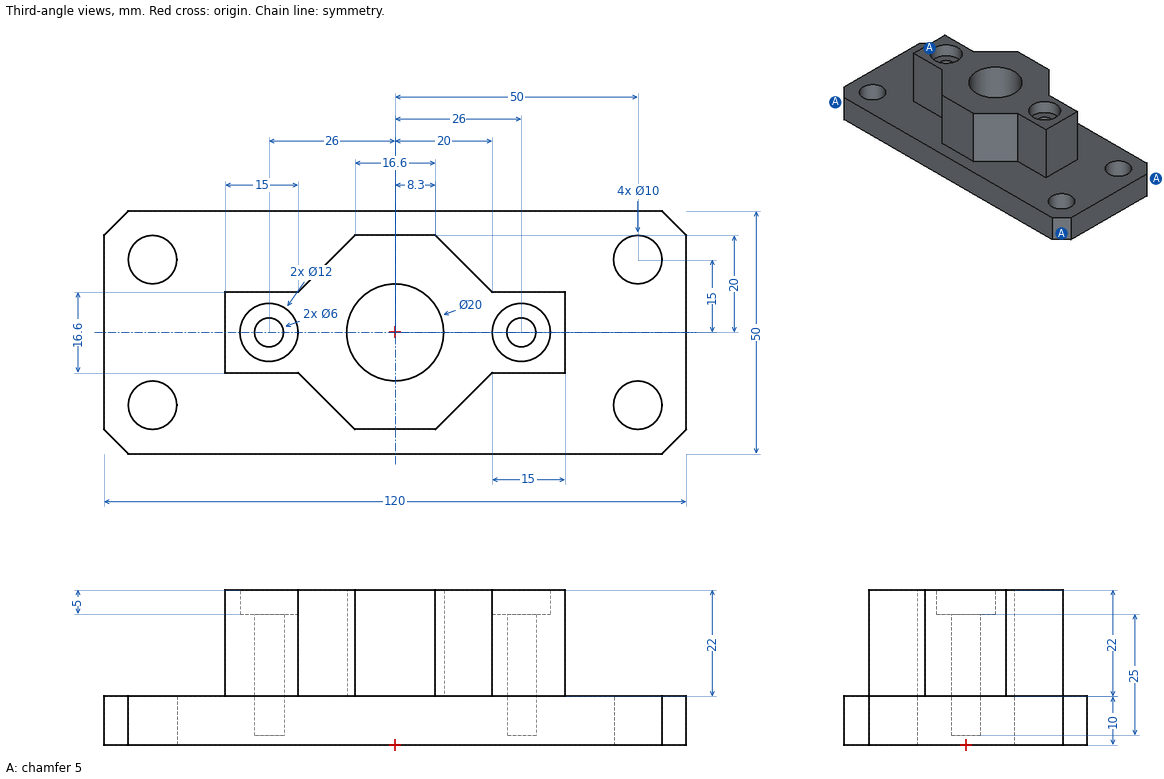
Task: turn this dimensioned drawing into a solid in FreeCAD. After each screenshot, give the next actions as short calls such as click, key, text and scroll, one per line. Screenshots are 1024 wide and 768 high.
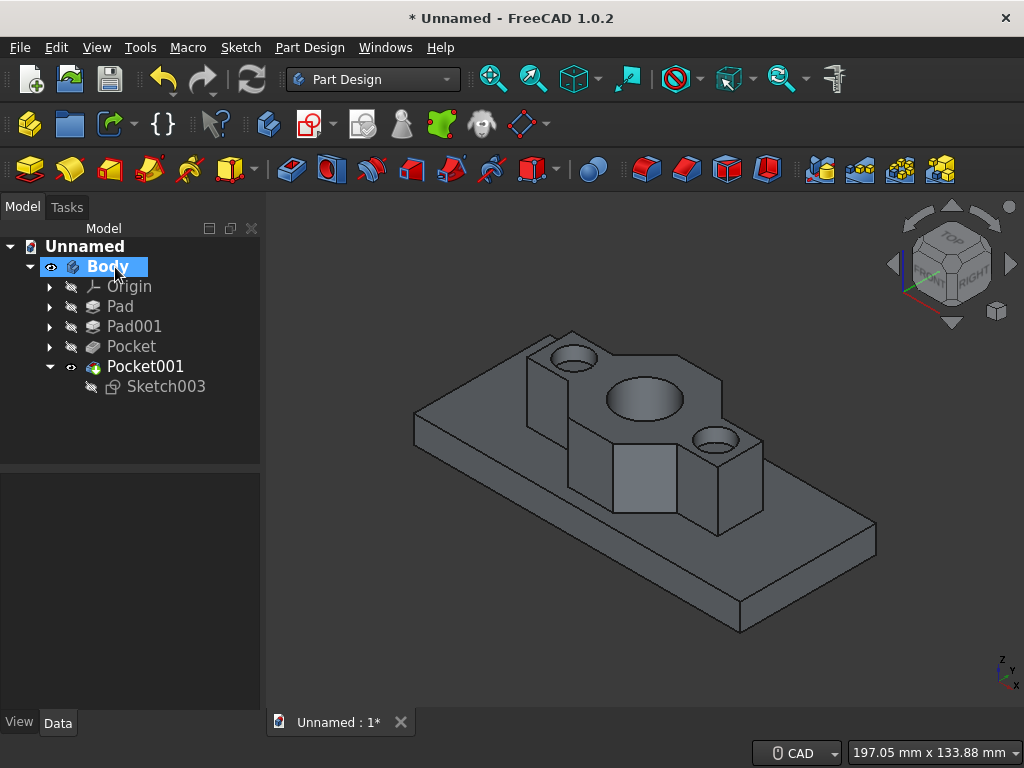
key(2)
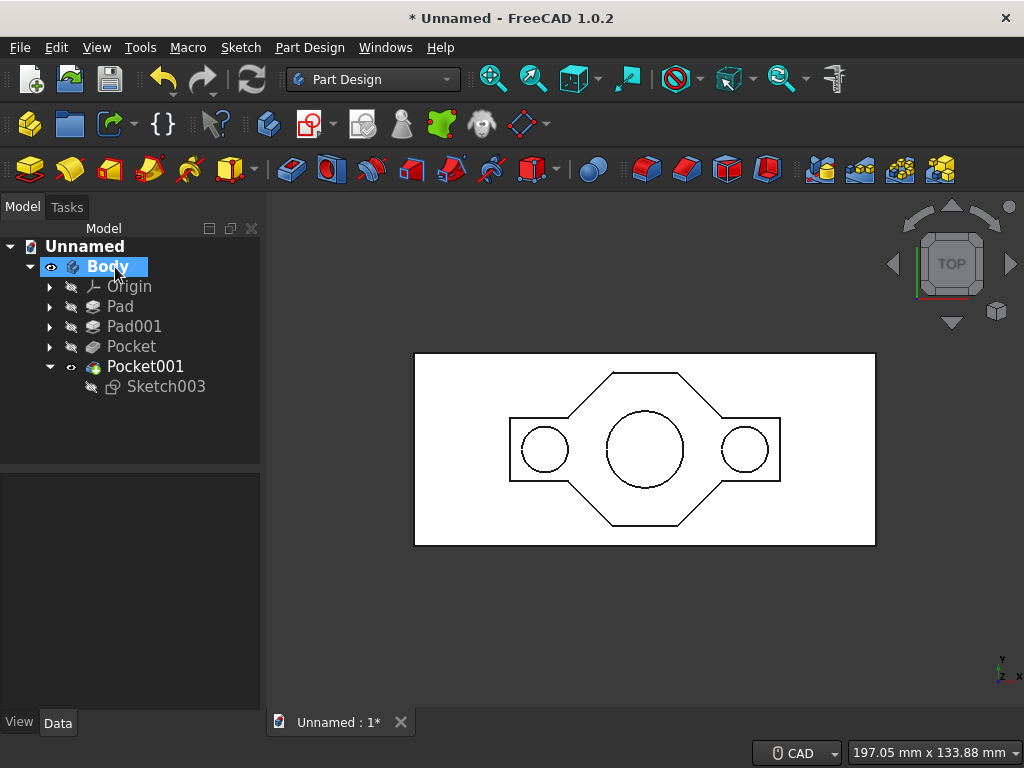
click(745, 449)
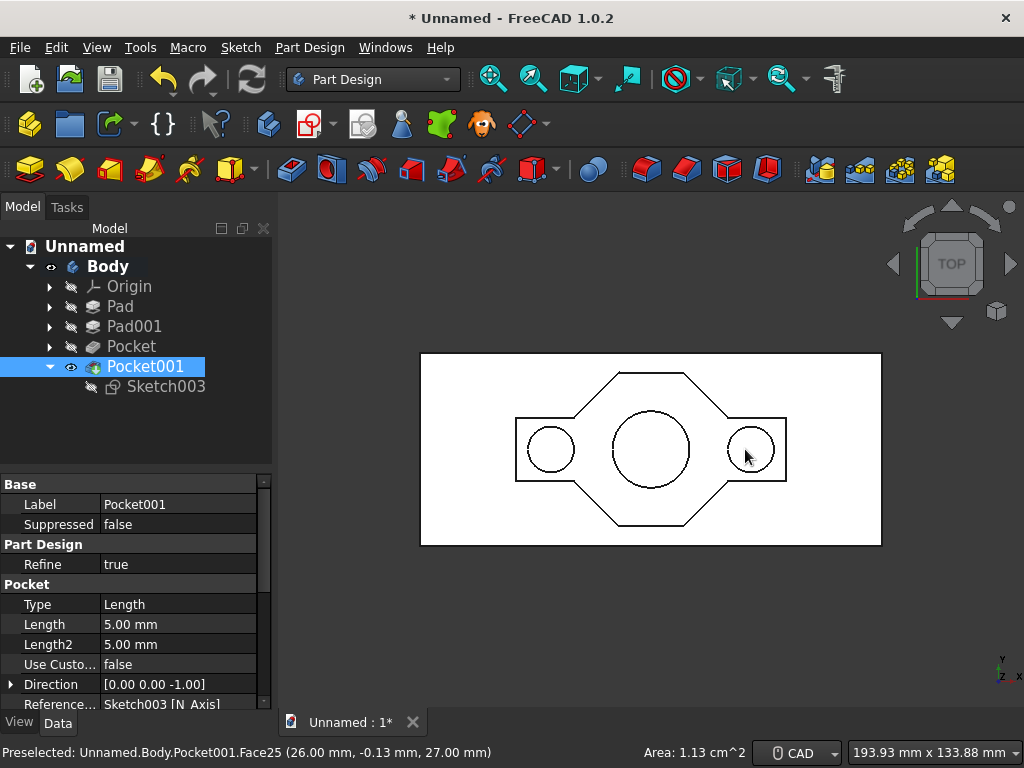
click(310, 124)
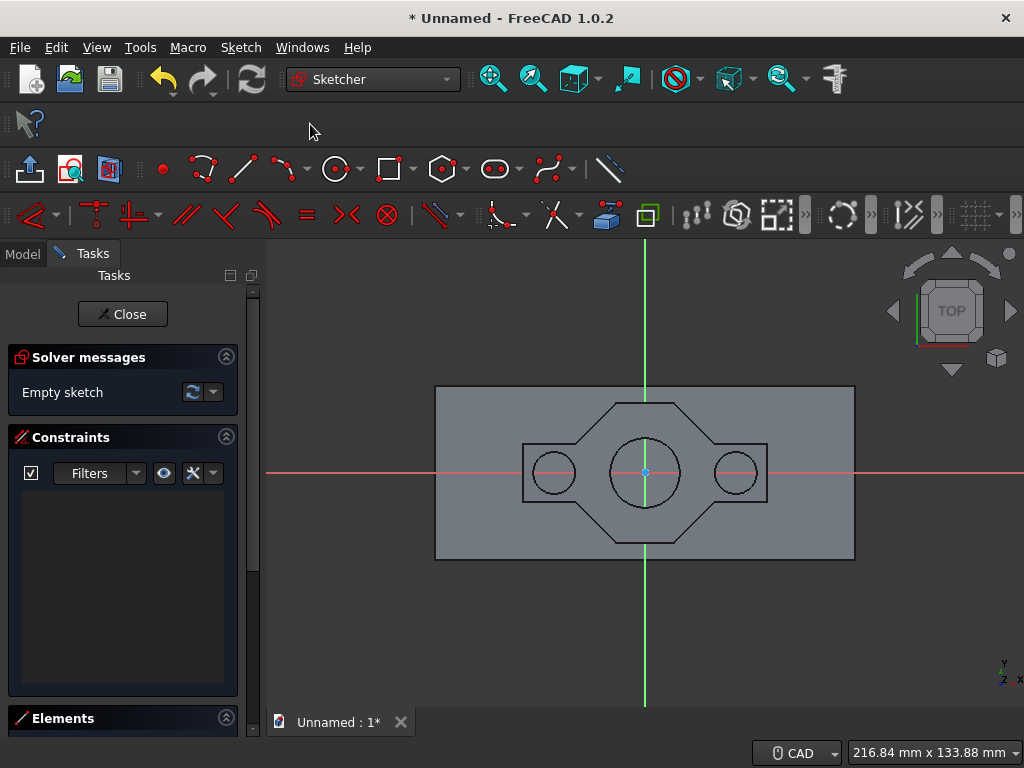
click(110, 170)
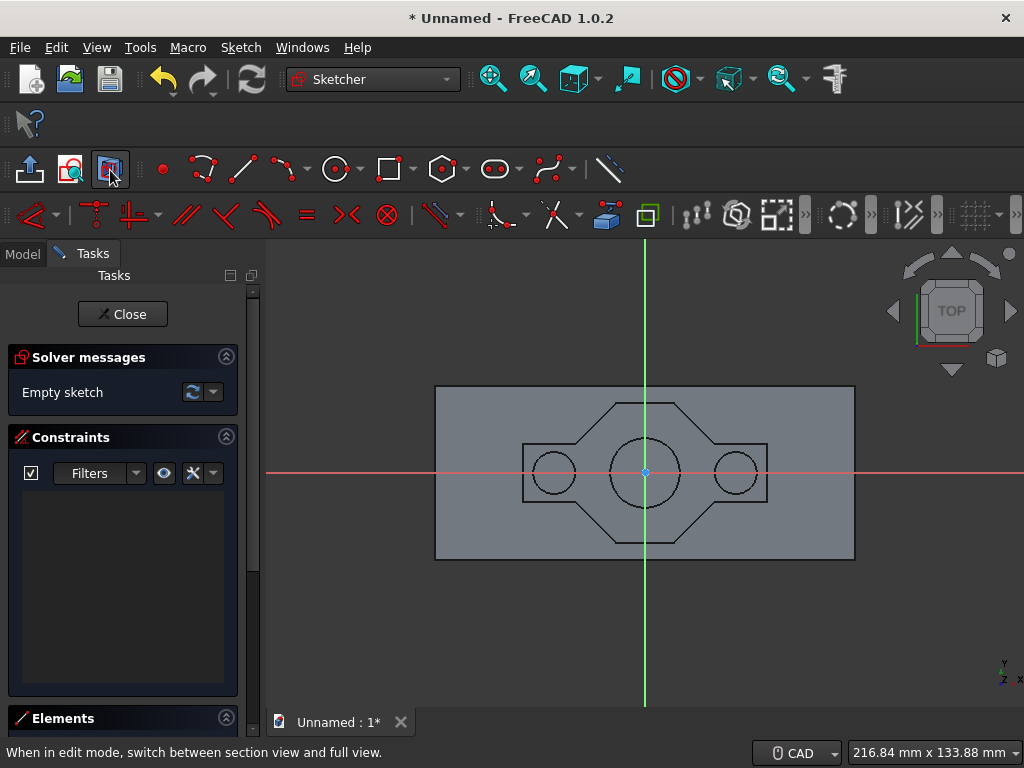
scroll(728, 473, up, 3)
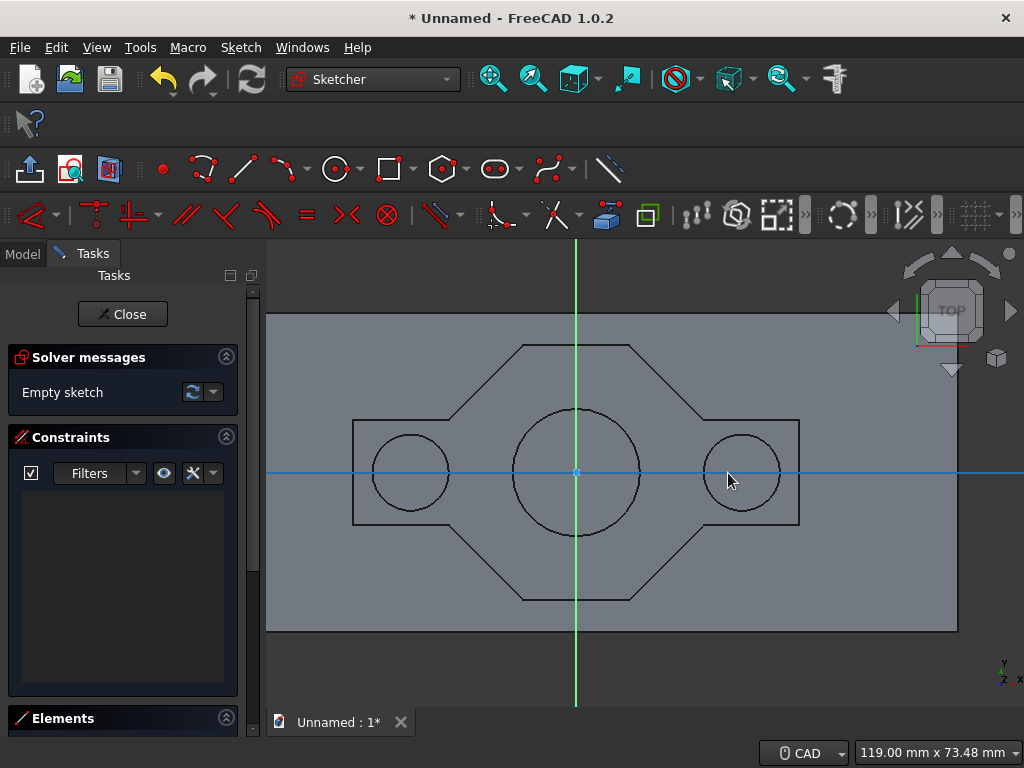
click(336, 170)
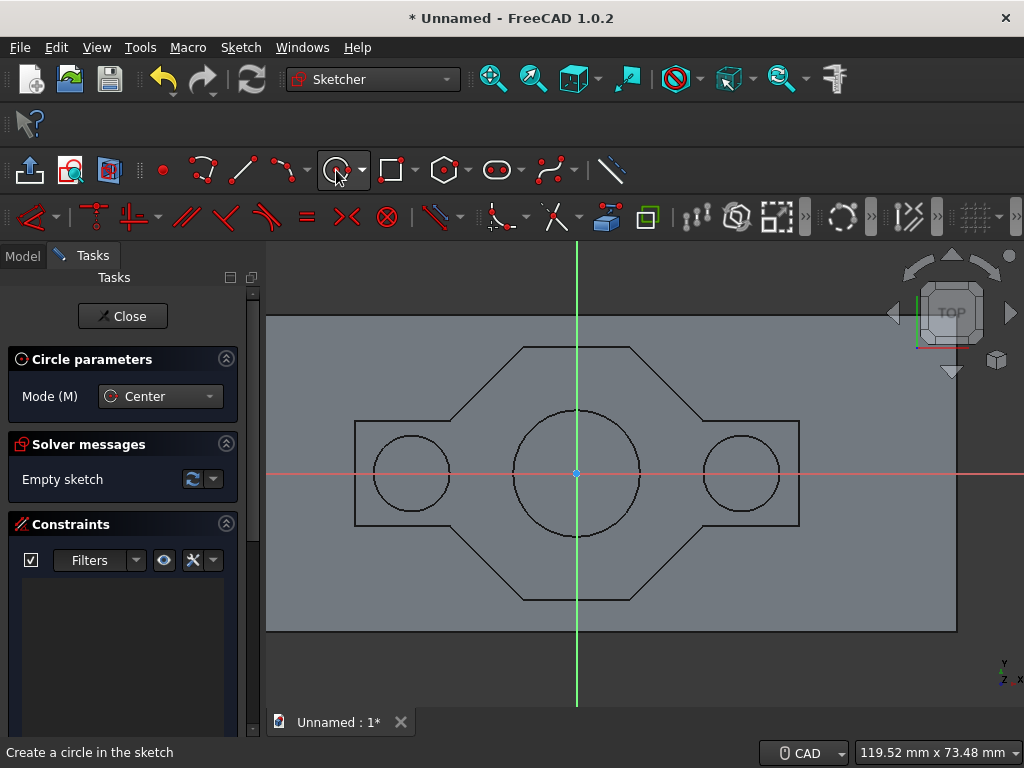
click(412, 474)
click(418, 456)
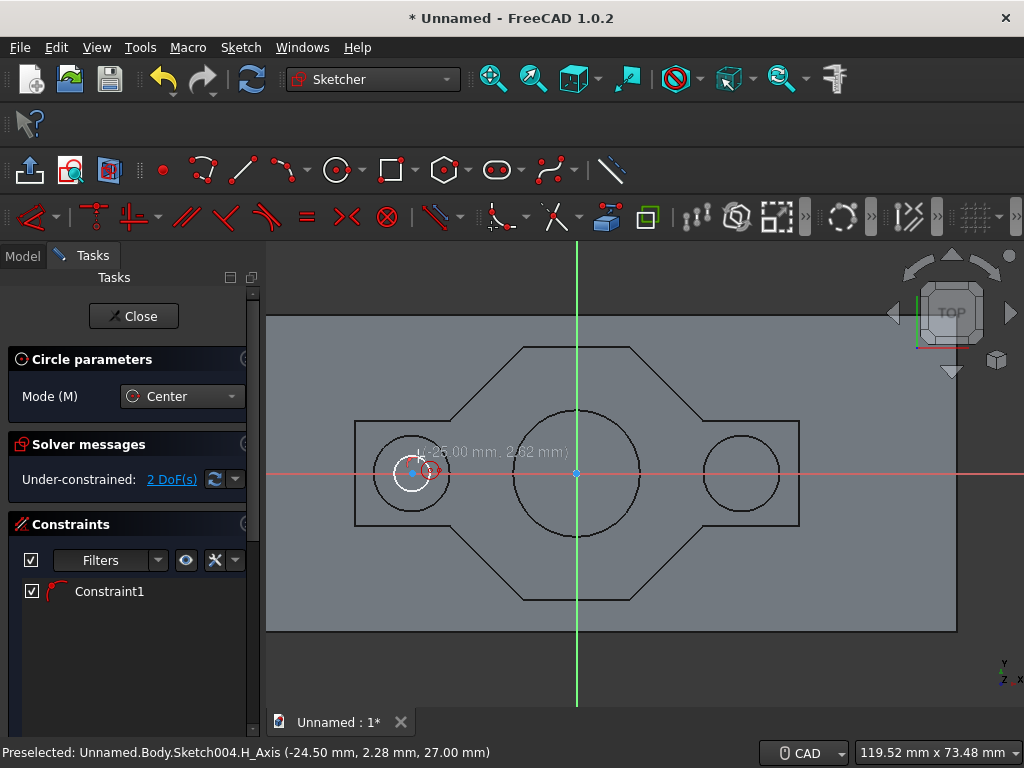
click(741, 474)
click(748, 456)
key(Escape)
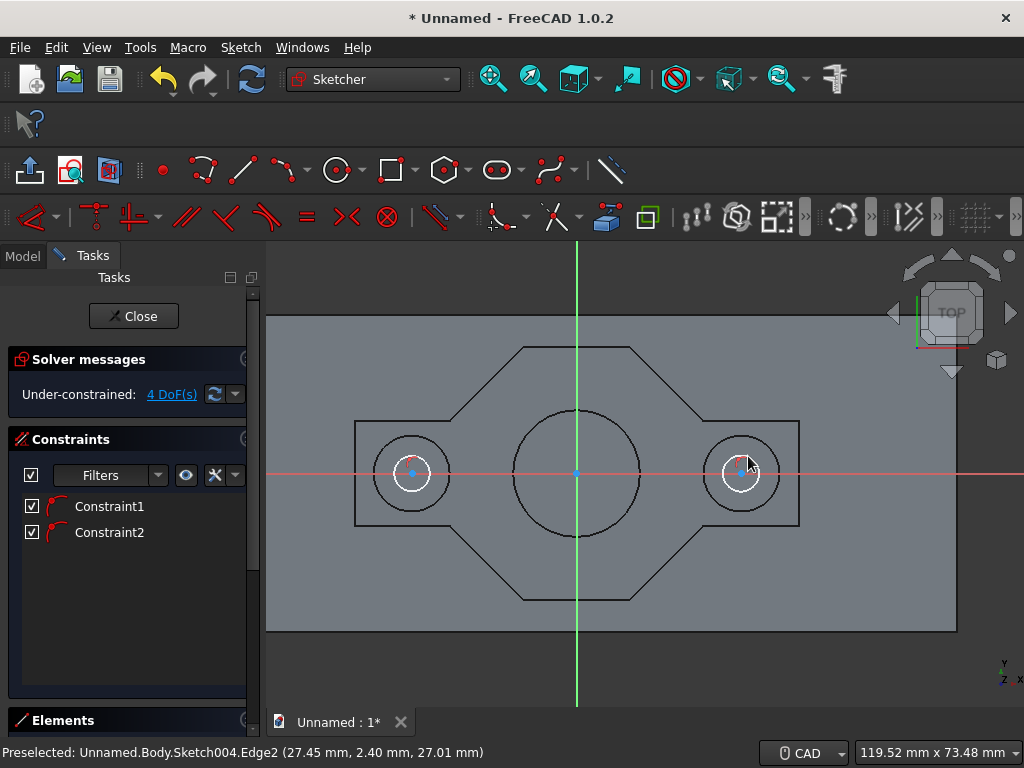
click(424, 461)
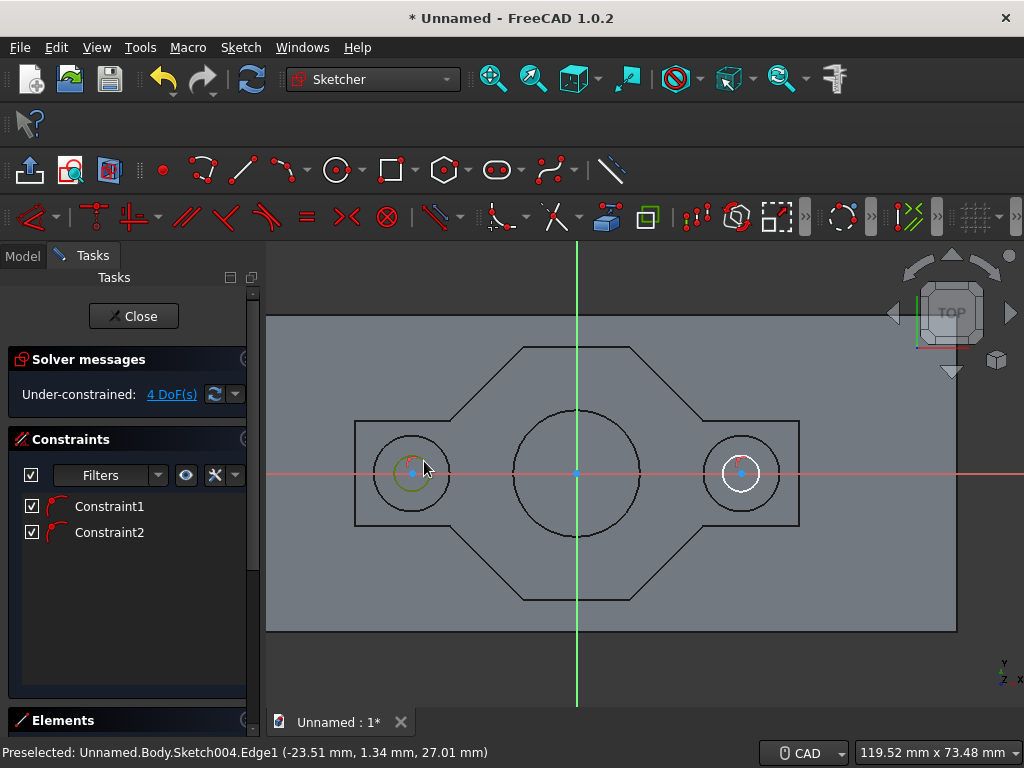
click(754, 461)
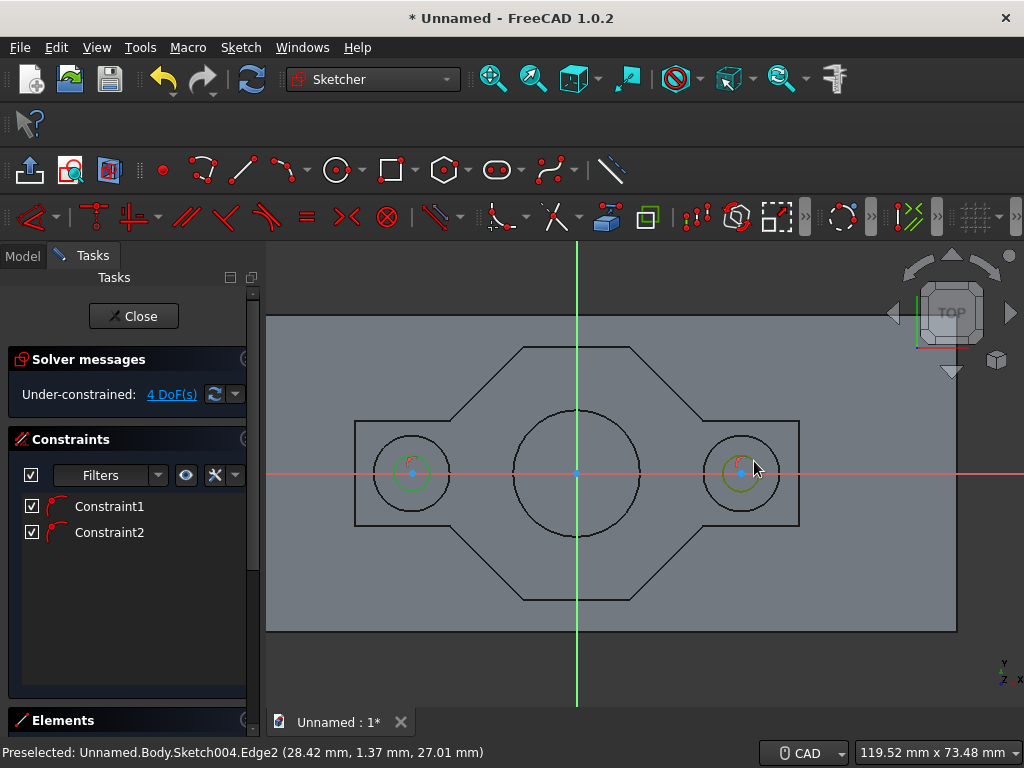
click(308, 218)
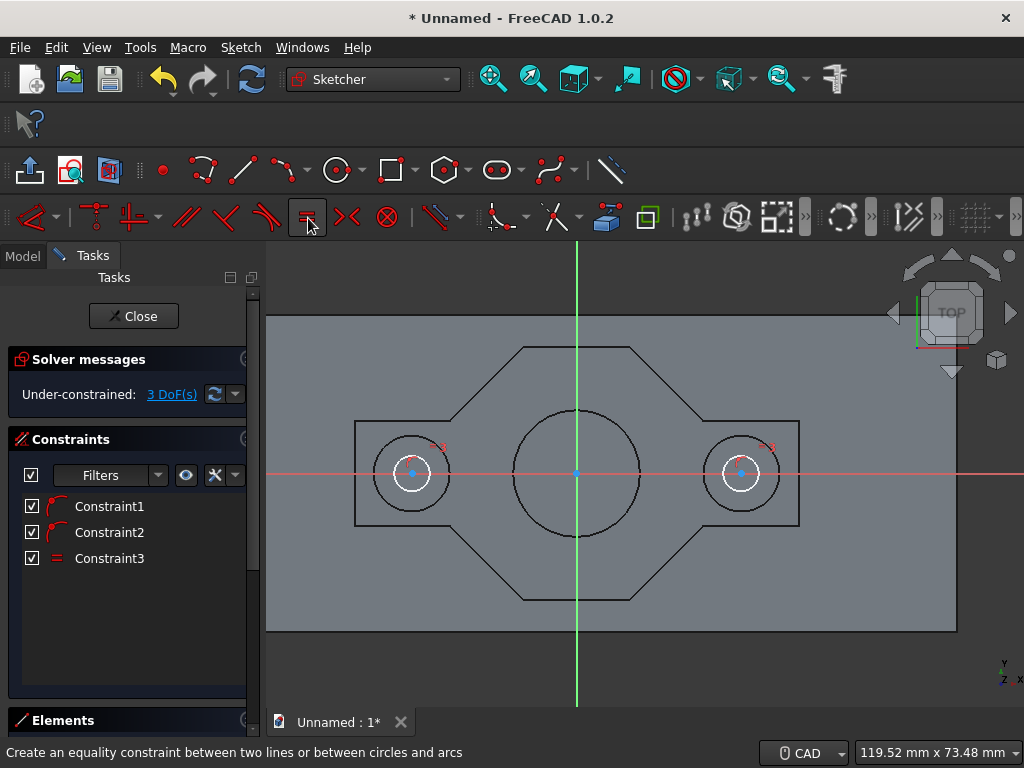
click(32, 218)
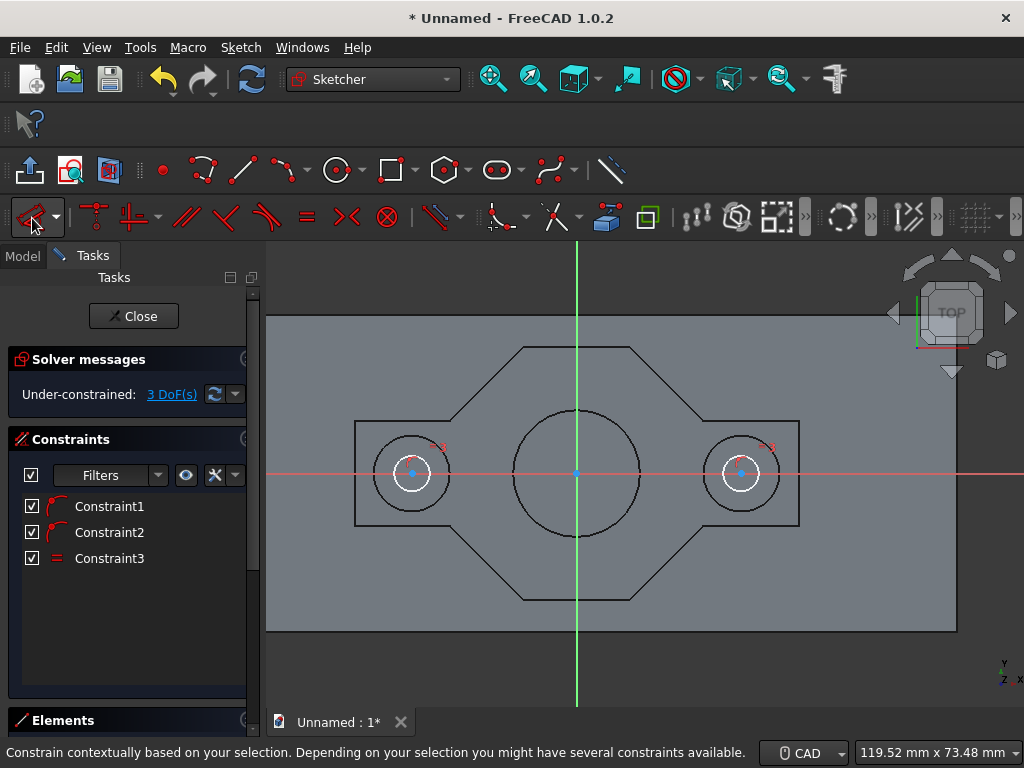
click(424, 461)
click(446, 438)